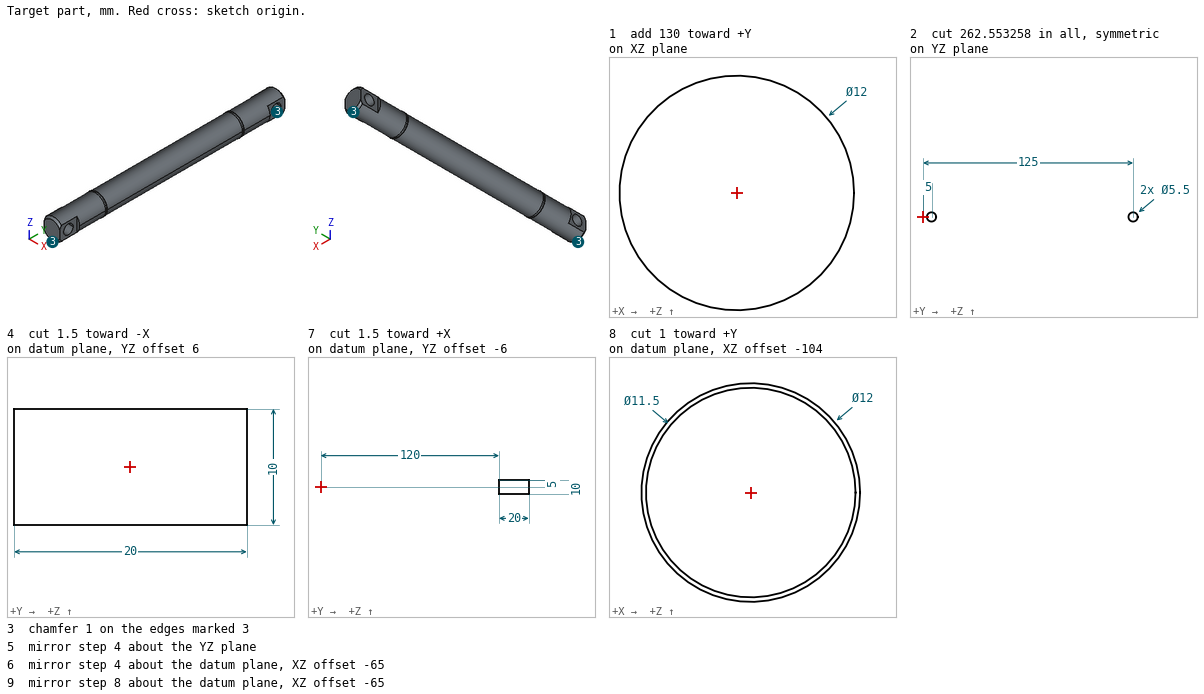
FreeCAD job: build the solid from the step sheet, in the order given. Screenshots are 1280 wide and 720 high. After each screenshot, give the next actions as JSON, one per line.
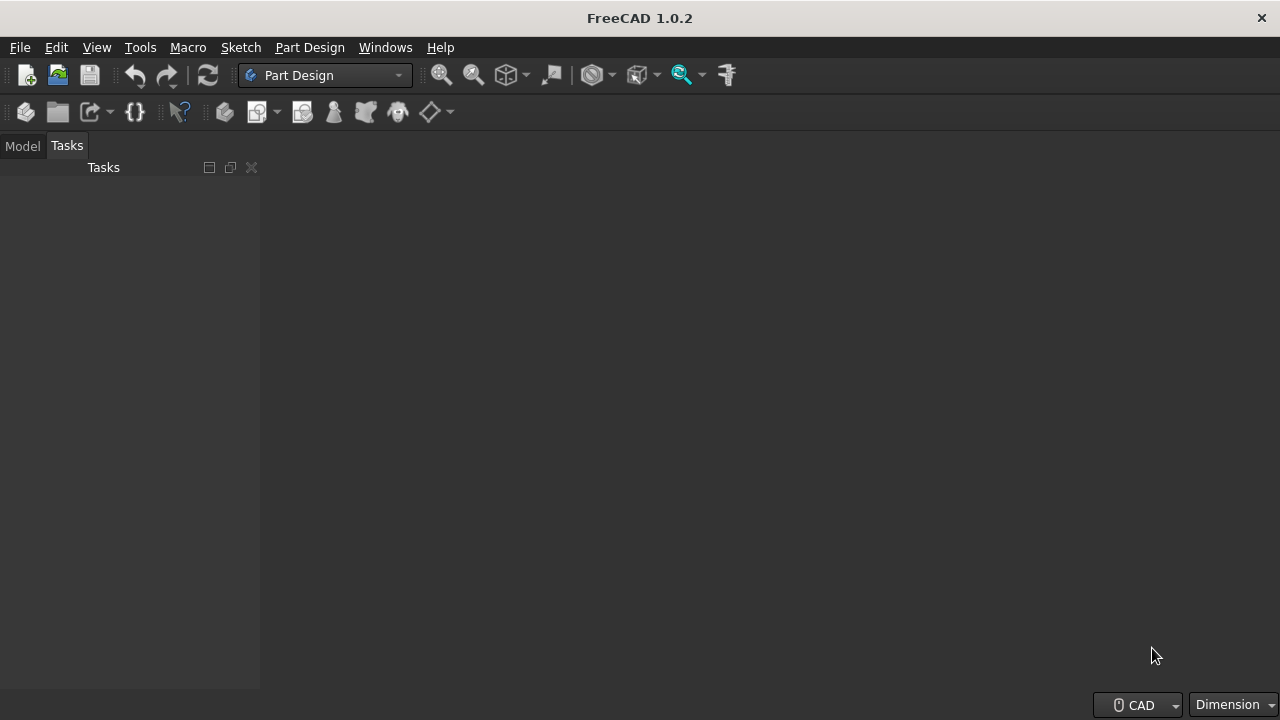
{"action": "left_click", "coordinate": [1100, 76]}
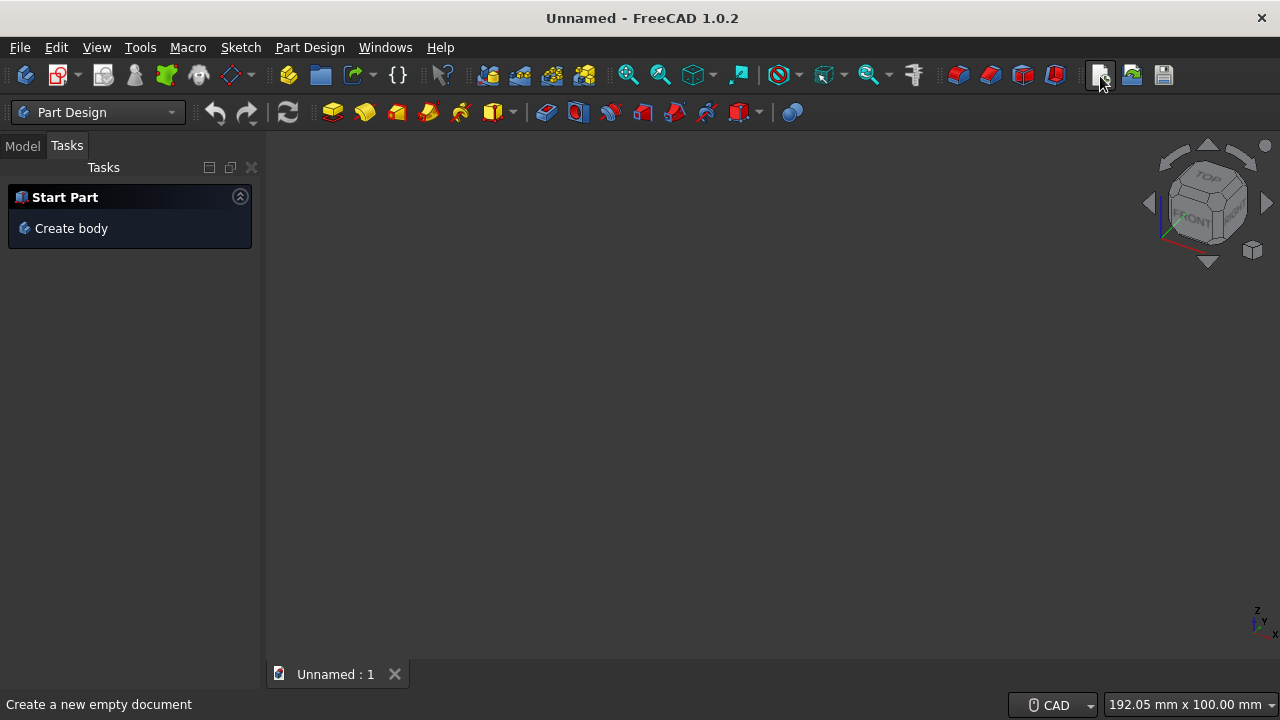
{"action": "left_click", "coordinate": [58, 76]}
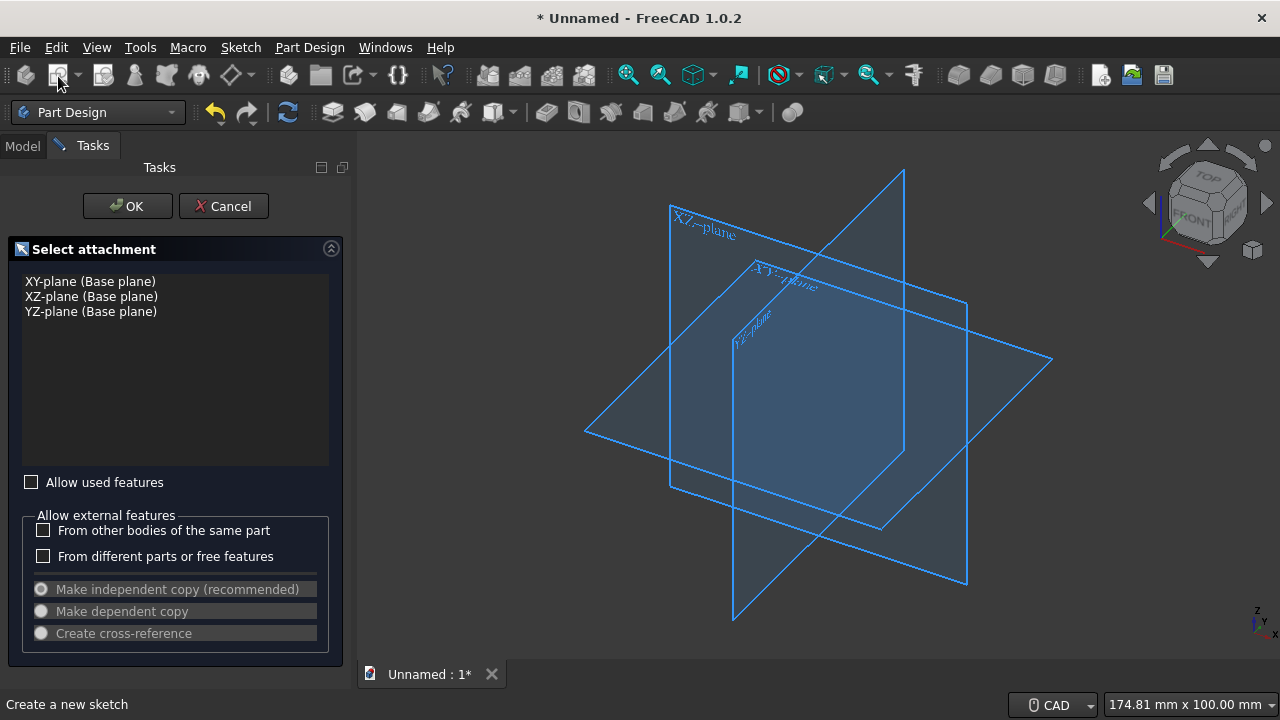
{"action": "left_click", "coordinate": [82, 296]}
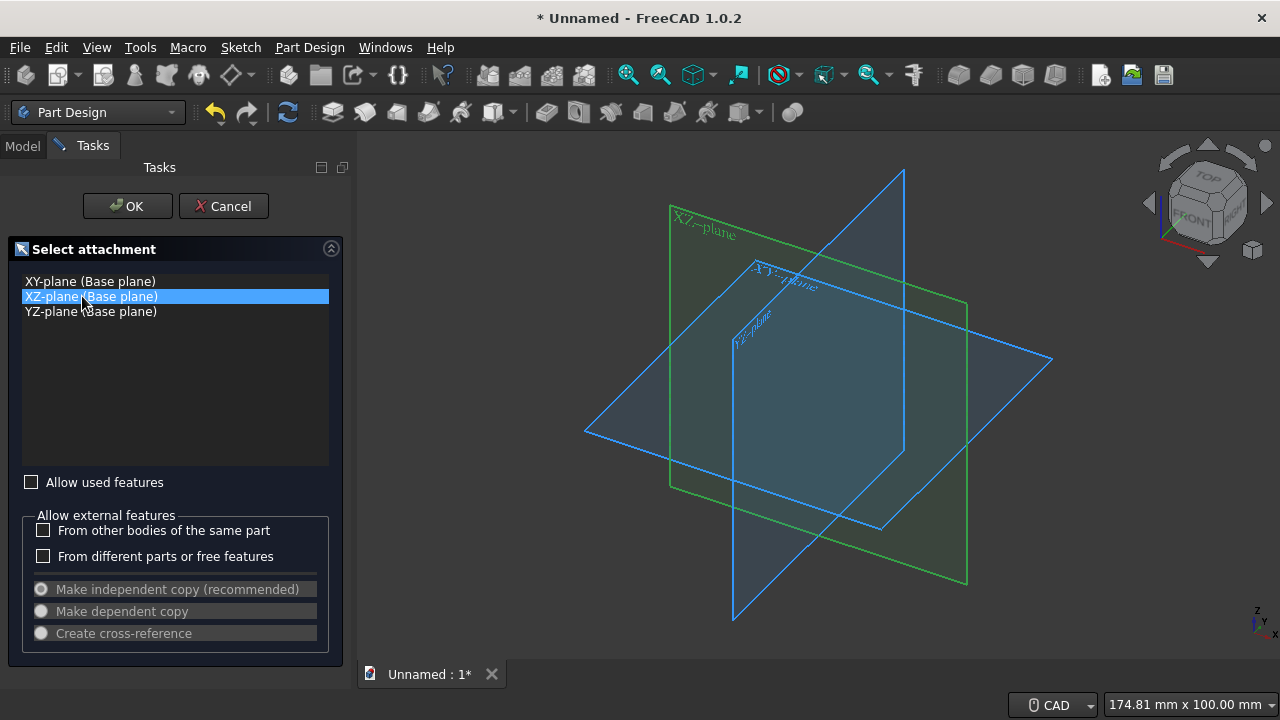
{"action": "left_click", "coordinate": [128, 206]}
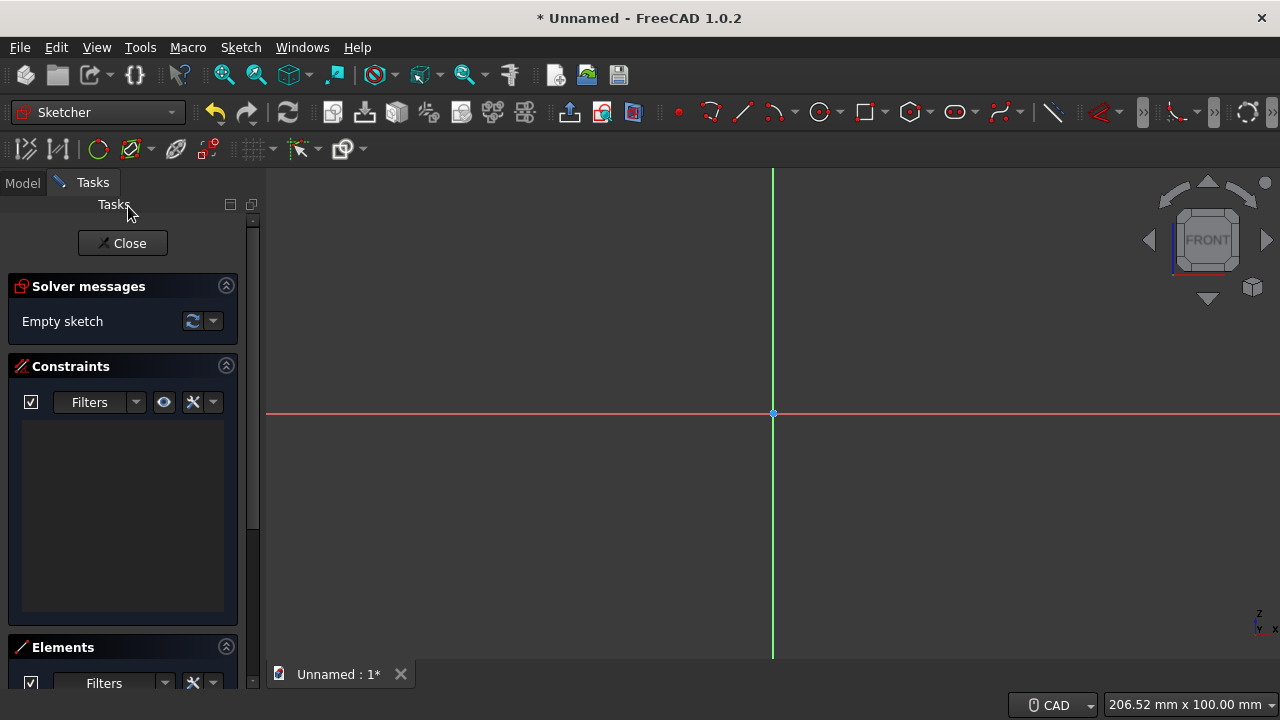
{"action": "scroll", "coordinate": [790, 414], "scroll_direction": "up", "scroll_amount": 8}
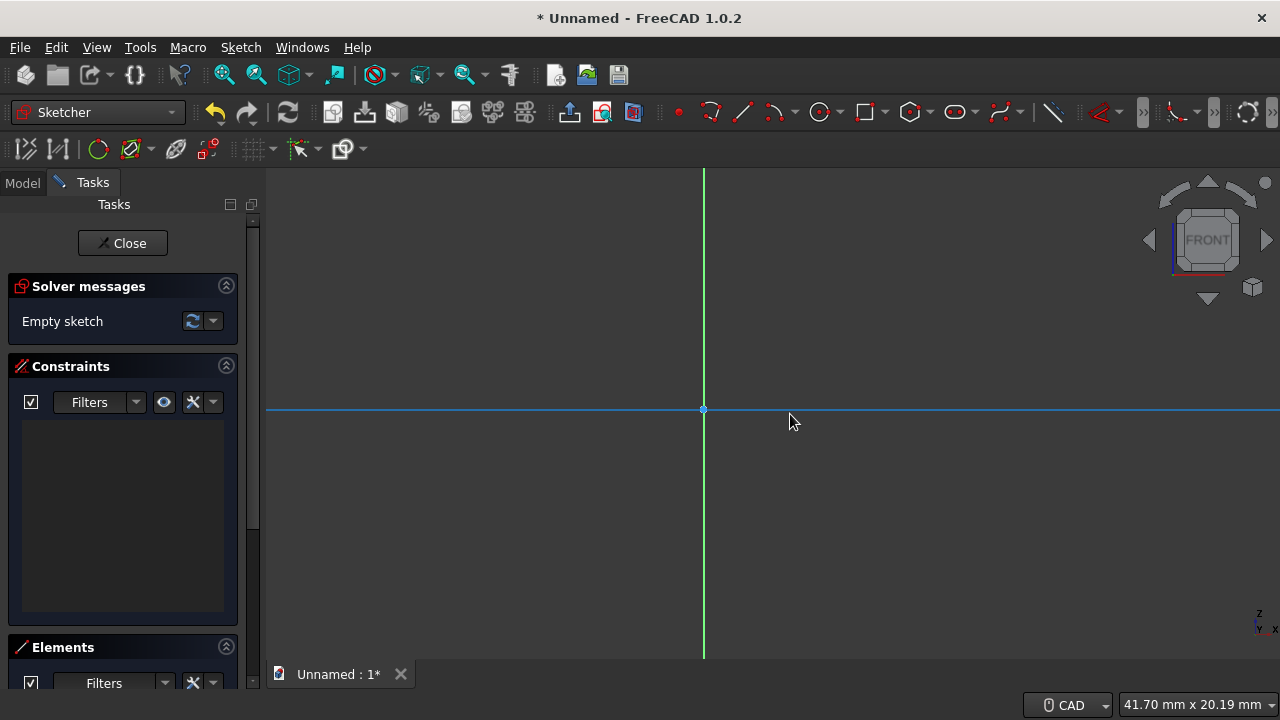
{"action": "key", "text": "g c"}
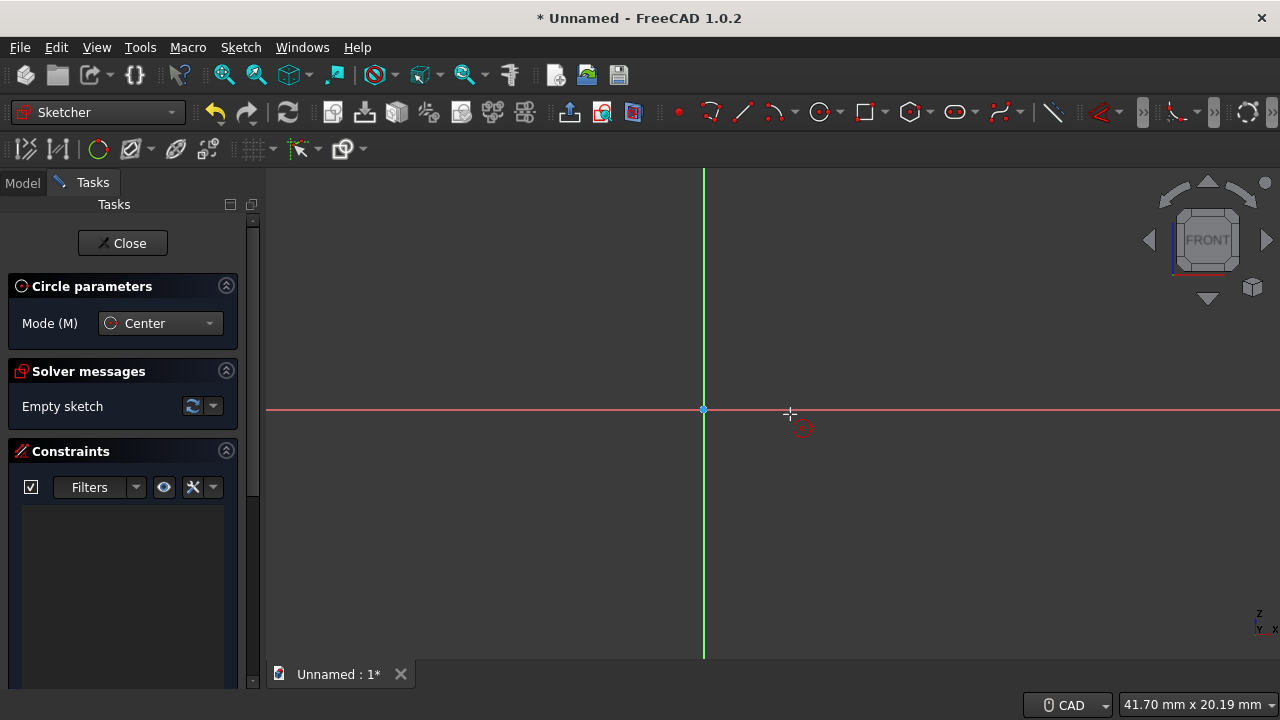
{"action": "left_click", "coordinate": [704, 410]}
{"action": "mouse_move", "coordinate": [807, 306]}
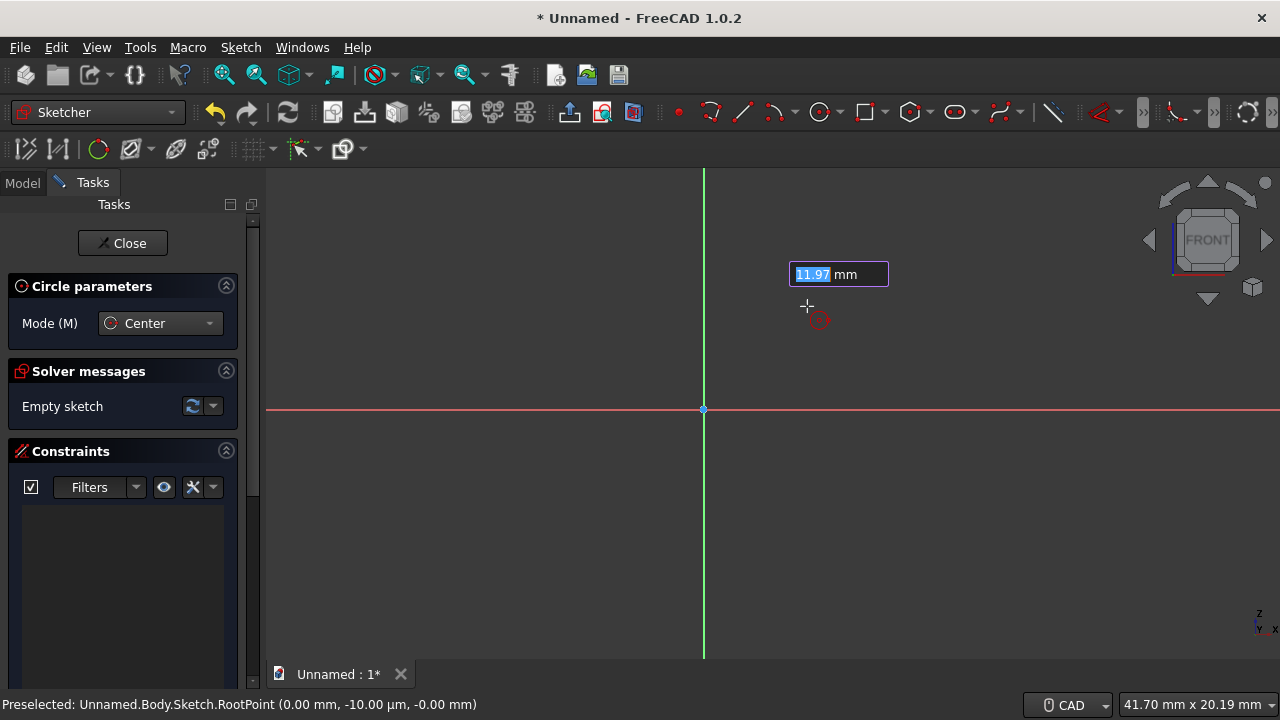
{"action": "type", "text": "12"}
{"action": "key", "text": "Return"}
{"action": "key", "text": "Escape"}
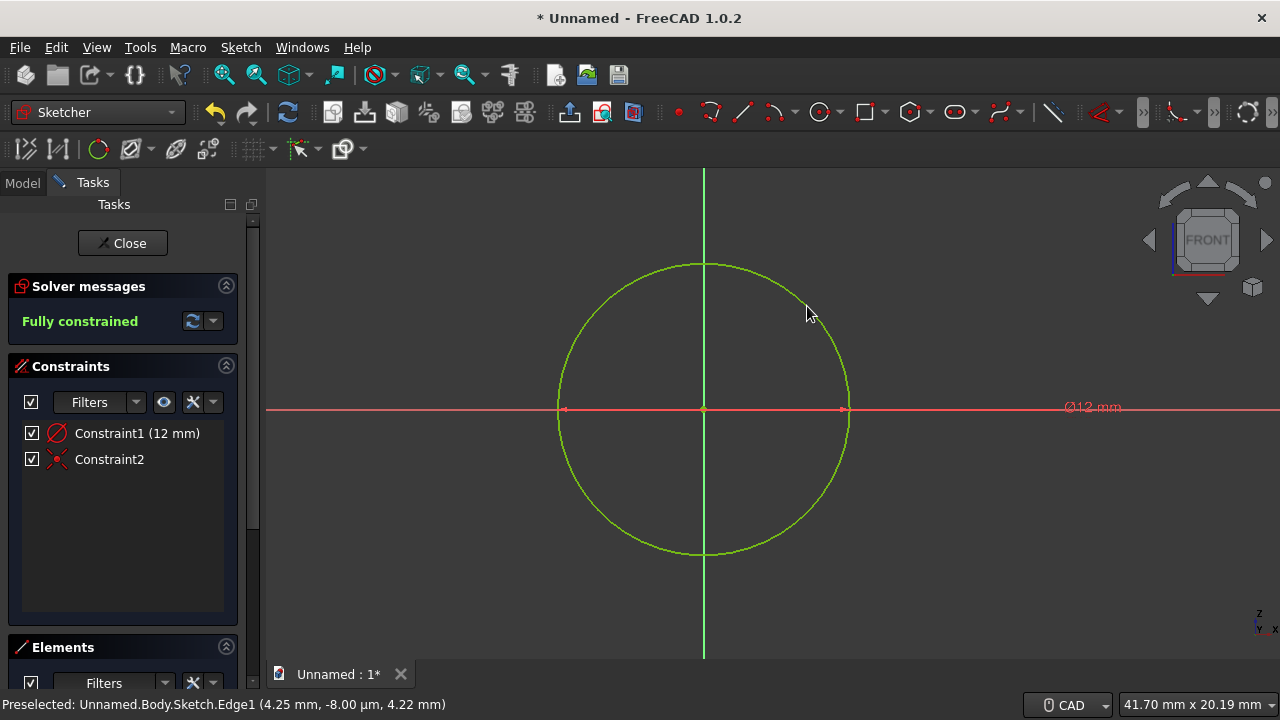
{"action": "left_click", "coordinate": [123, 243]}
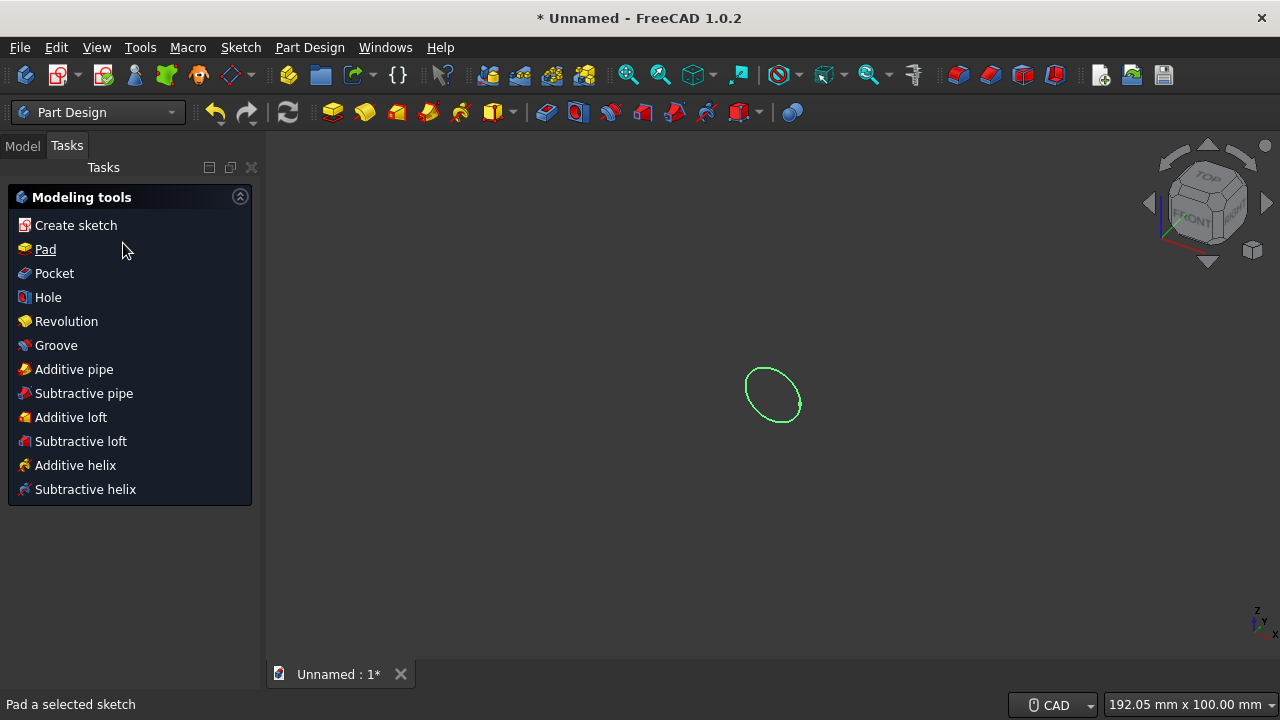
{"action": "left_click", "coordinate": [334, 112]}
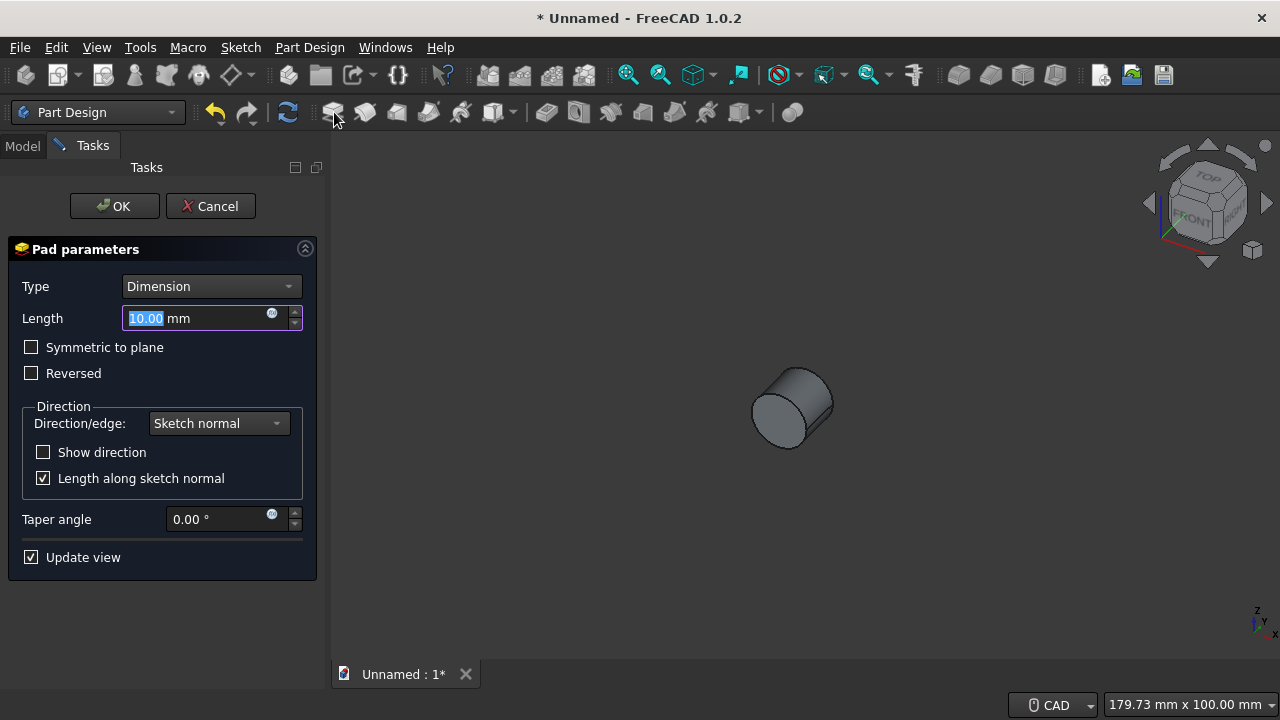
{"action": "type", "text": "130"}
{"action": "key", "text": "Tab"}